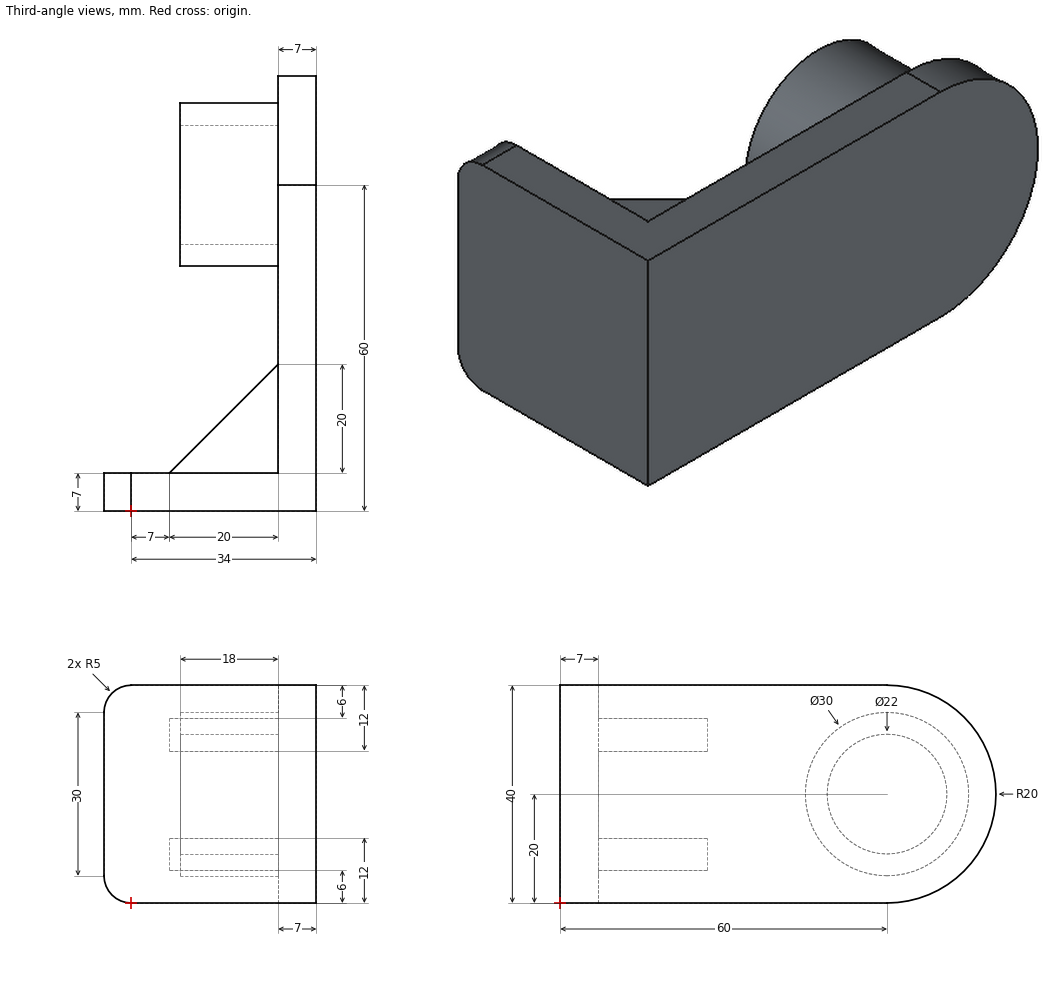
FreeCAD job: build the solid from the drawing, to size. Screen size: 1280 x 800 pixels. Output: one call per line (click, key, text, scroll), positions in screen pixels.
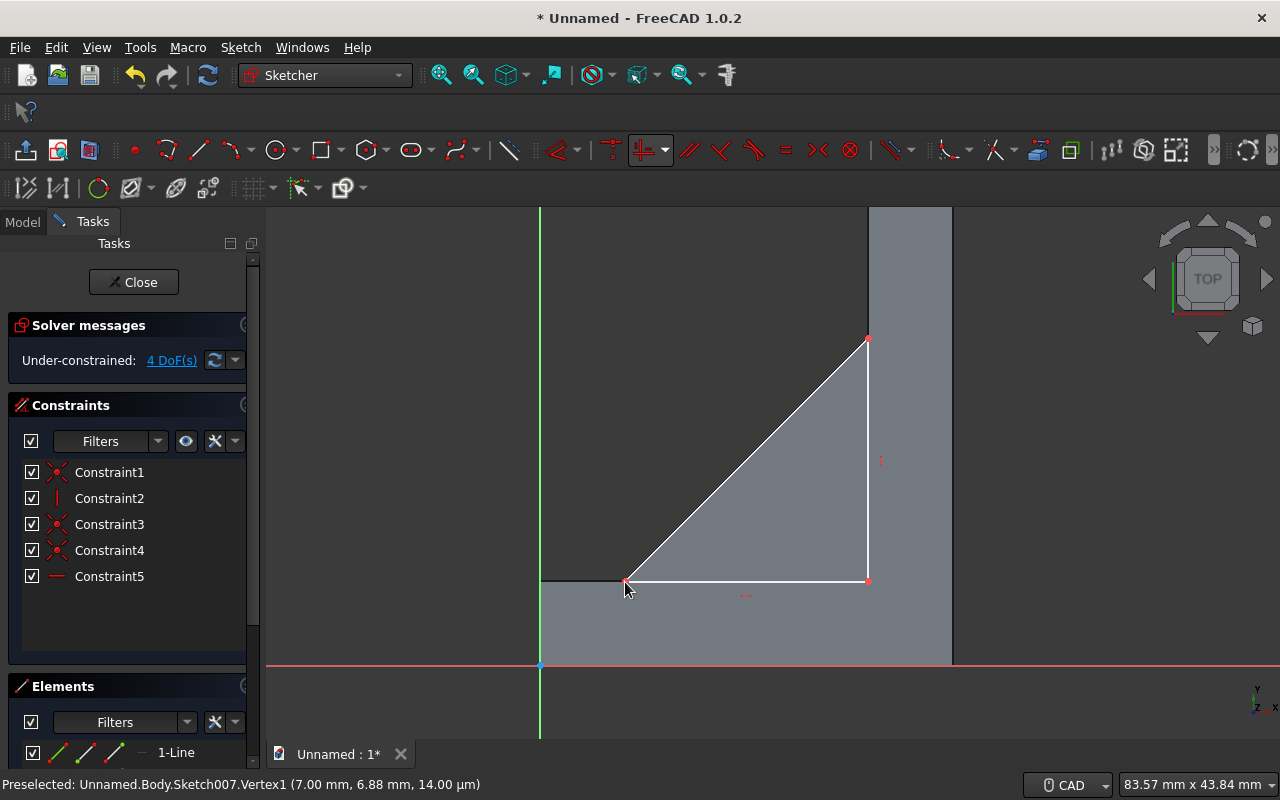
click(556, 150)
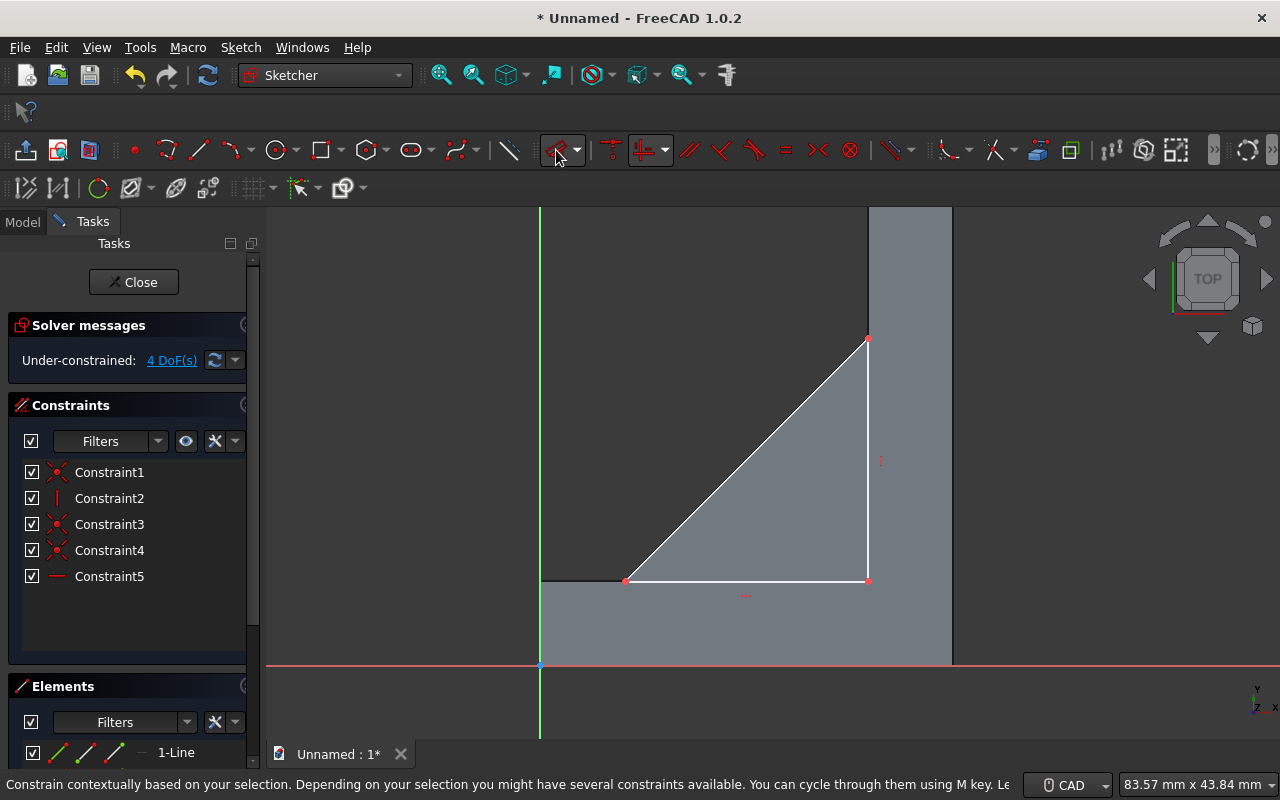
click(868, 412)
click(902, 461)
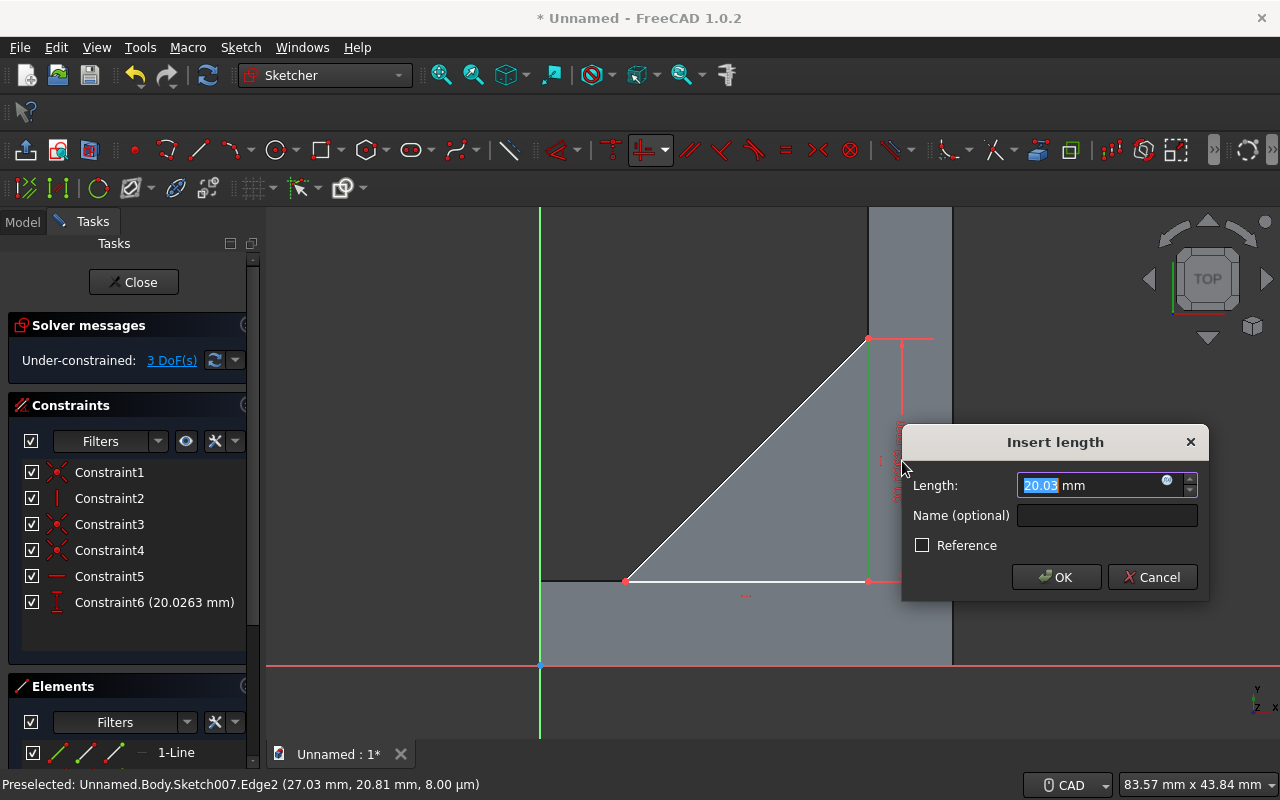
text(20)
key(Return)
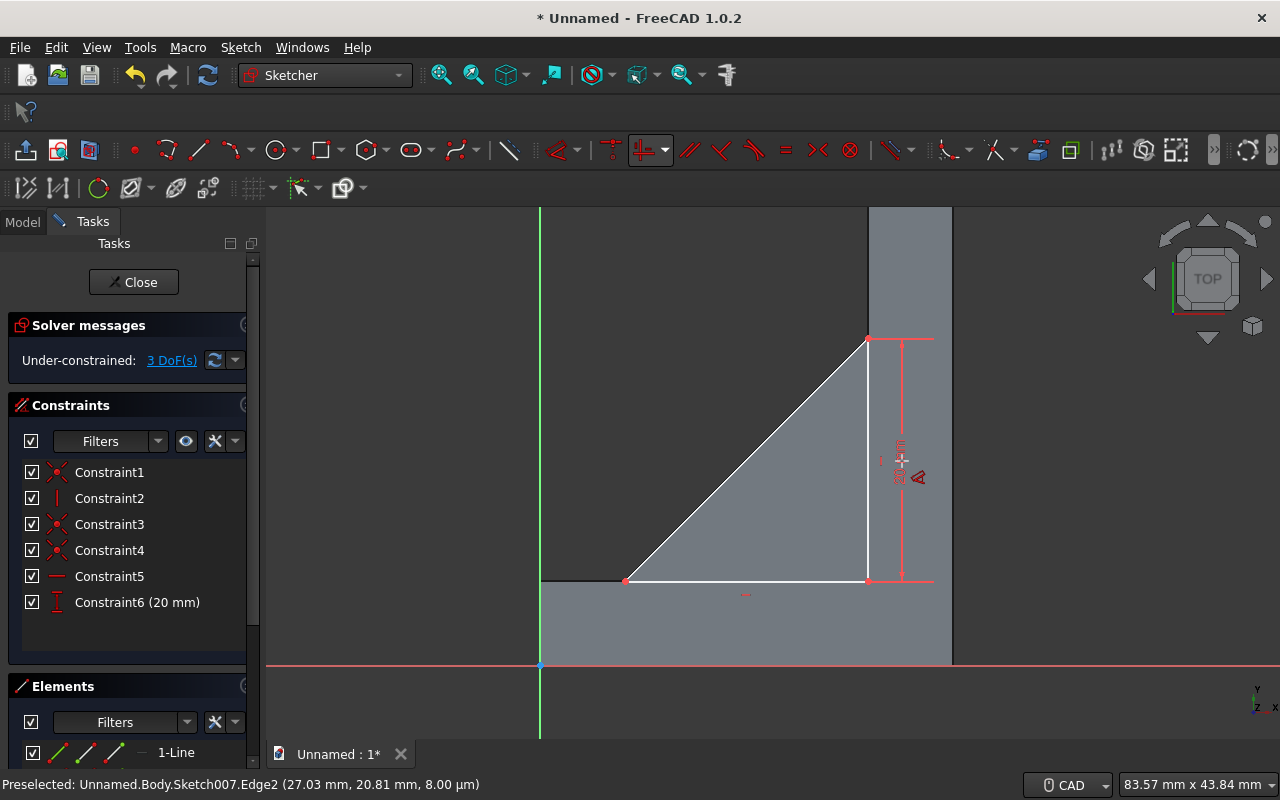
click(795, 582)
click(747, 616)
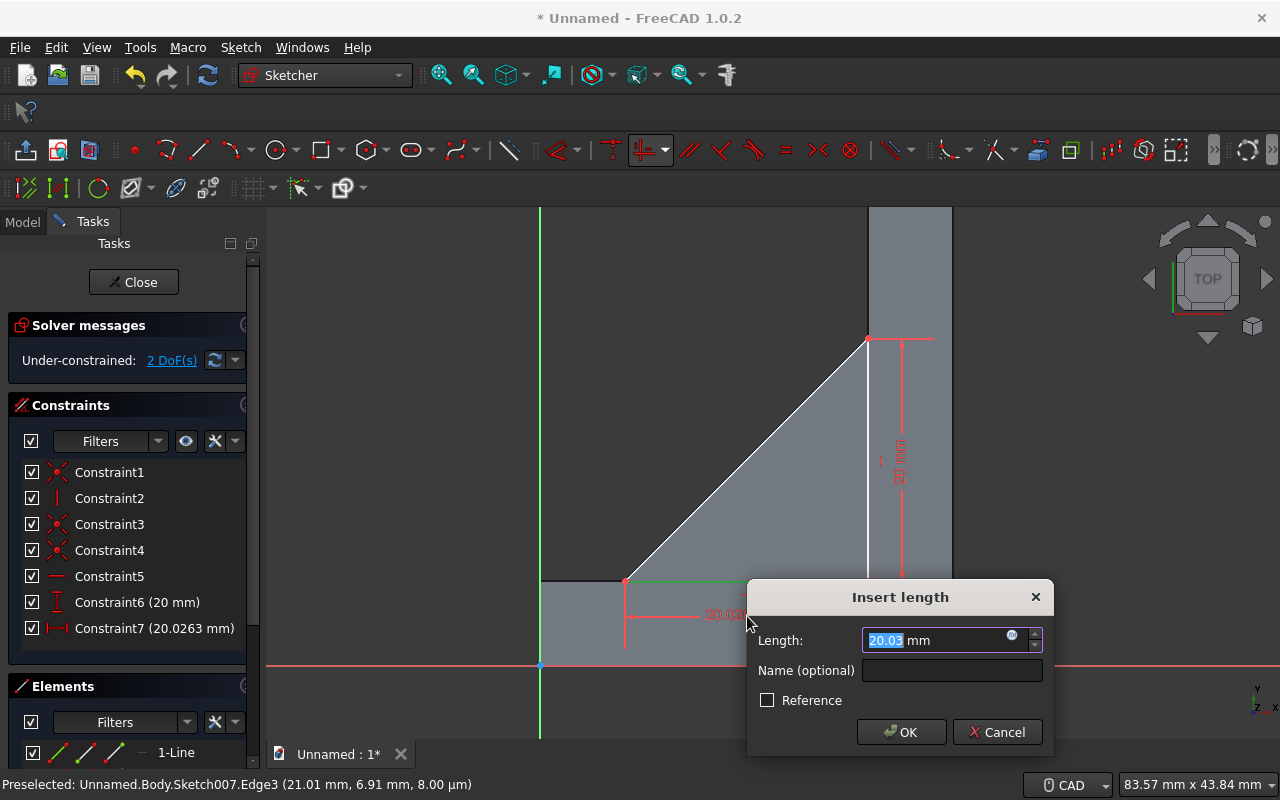
text(20)
key(Return)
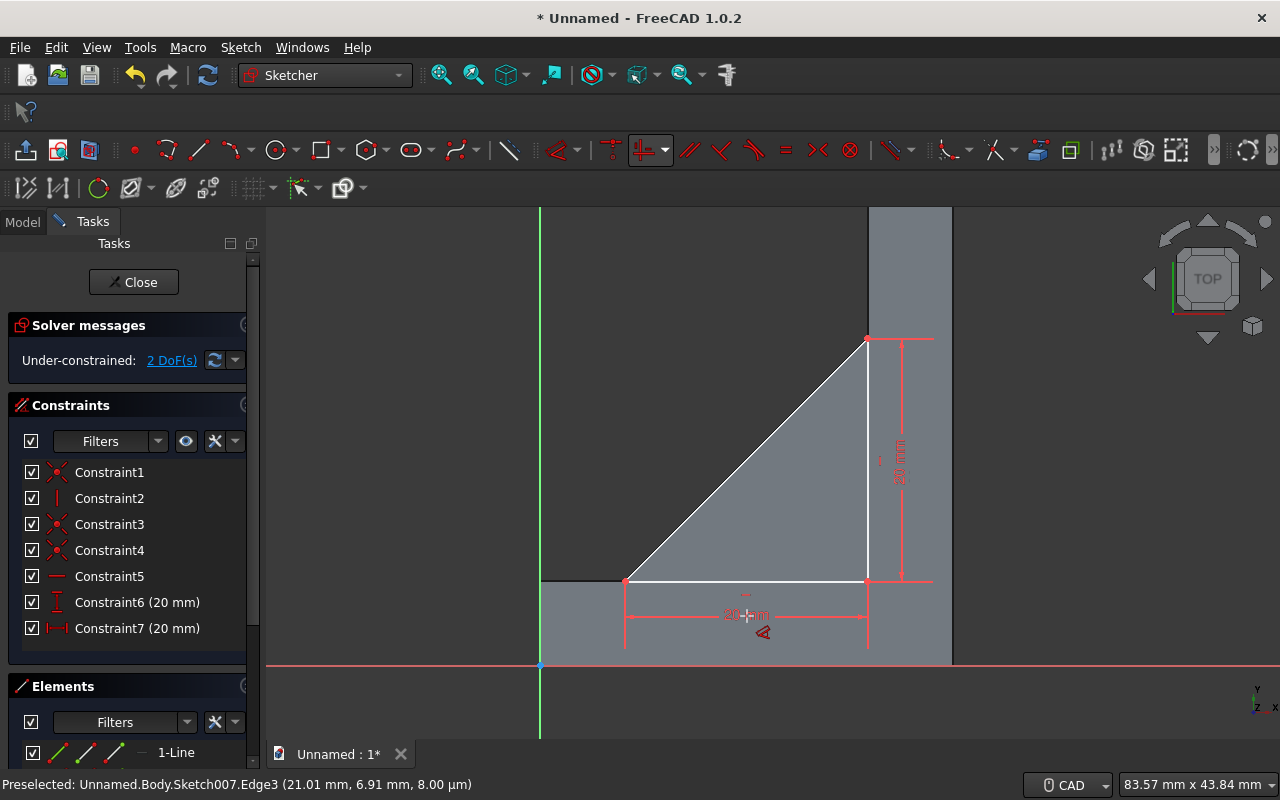
click(625, 582)
click(583, 700)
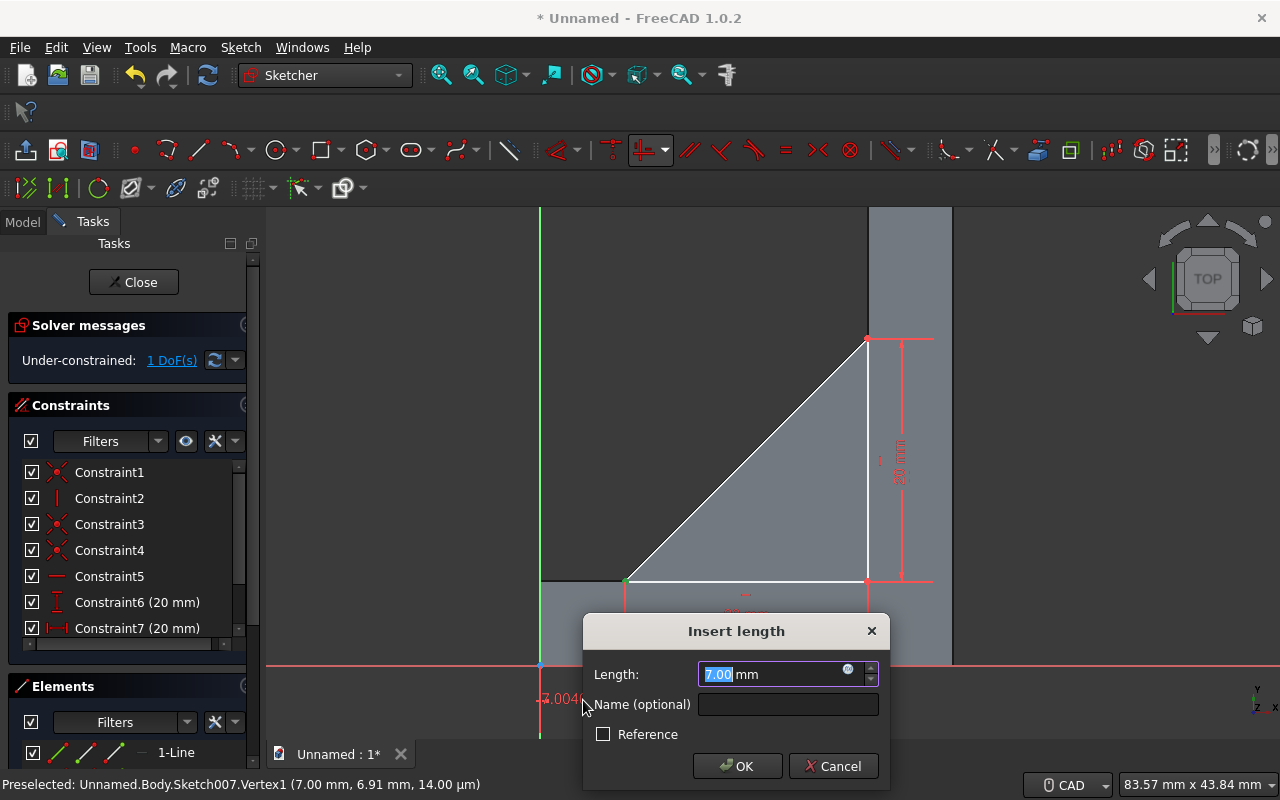
text(7)
key(Return)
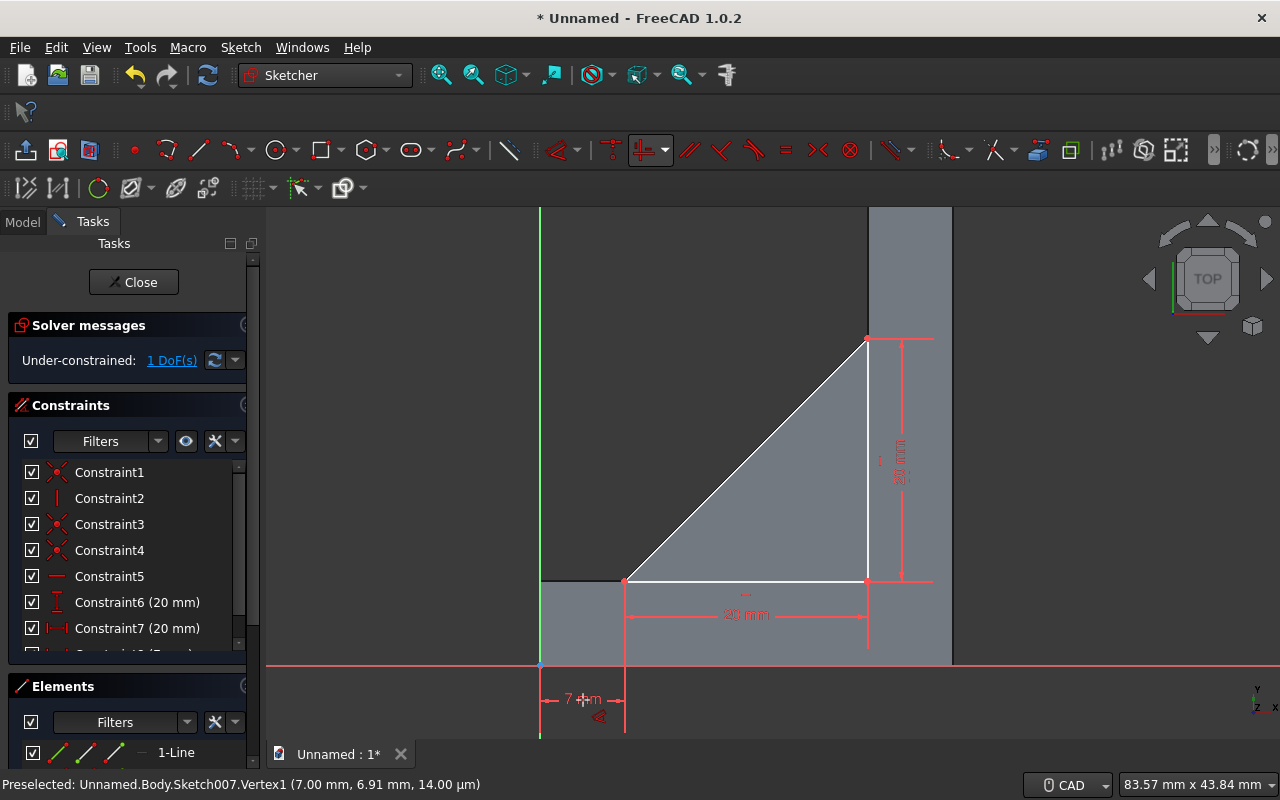
click(625, 582)
click(506, 624)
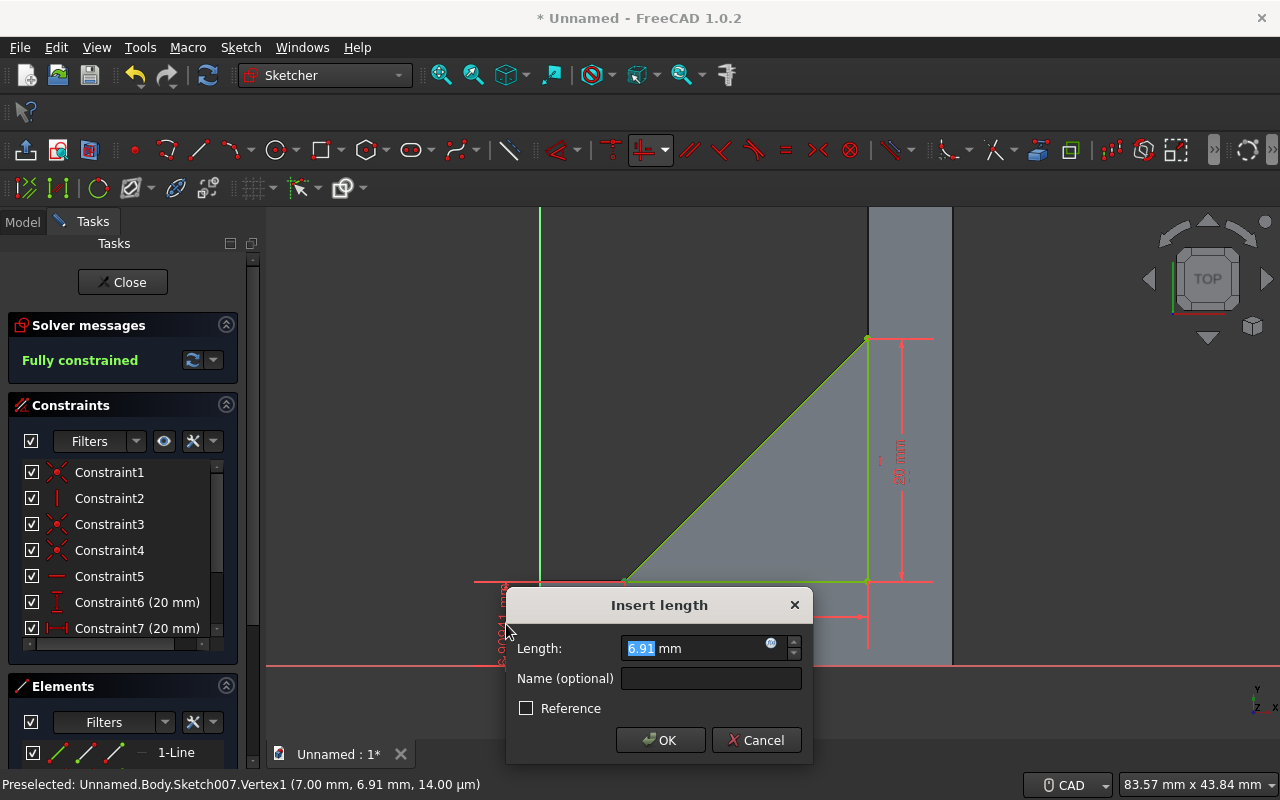
text(7)
key(Return)
key(Escape)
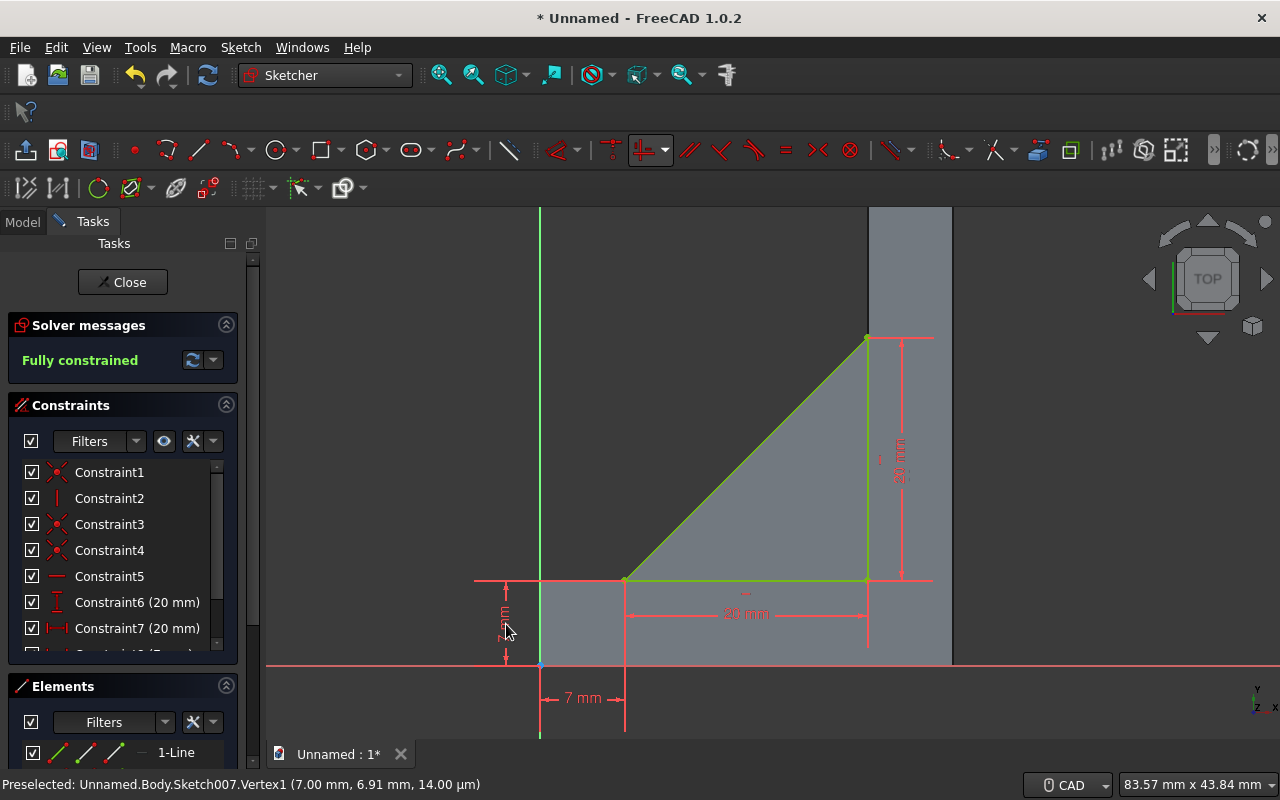
click(123, 282)